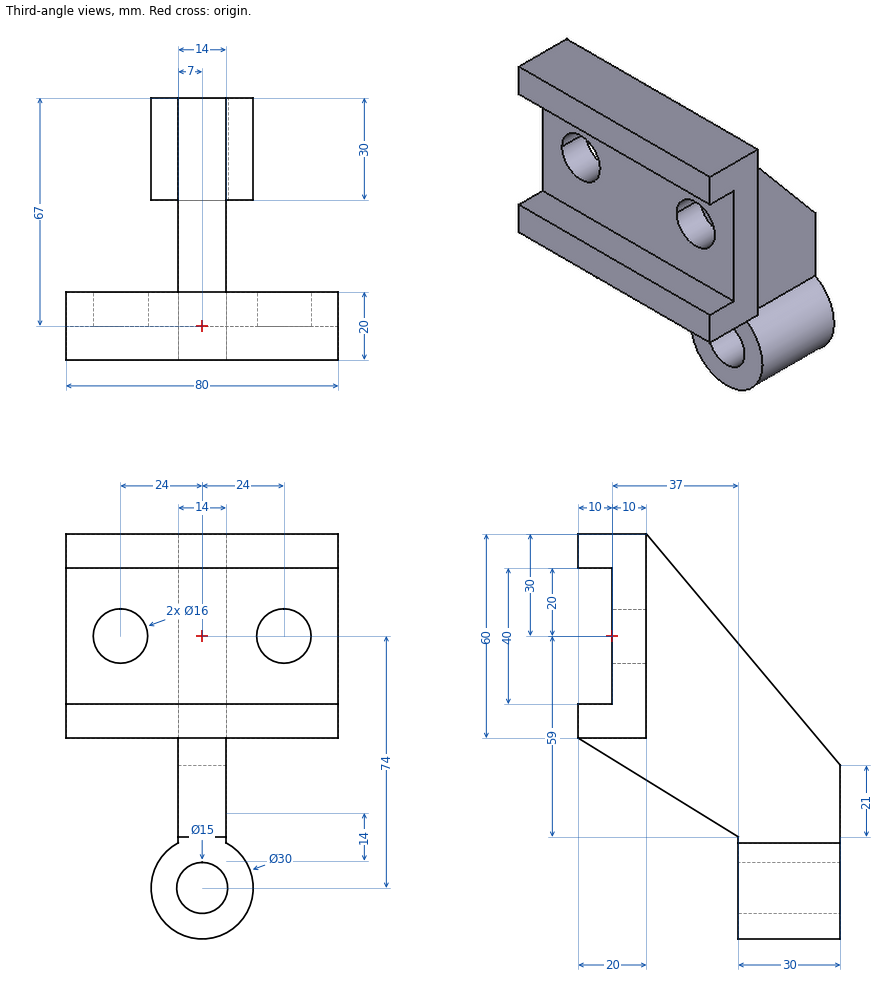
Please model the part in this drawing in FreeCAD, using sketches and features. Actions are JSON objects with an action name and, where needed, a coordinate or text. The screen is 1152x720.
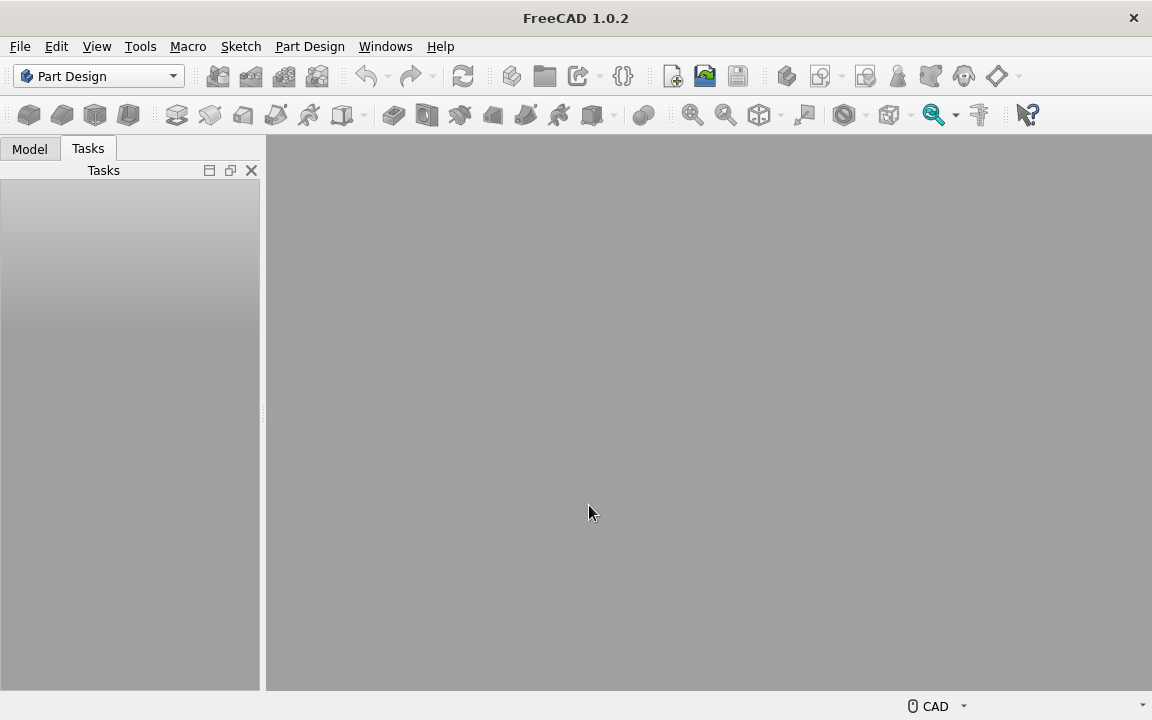
{"action": "left_click", "coordinate": [672, 76]}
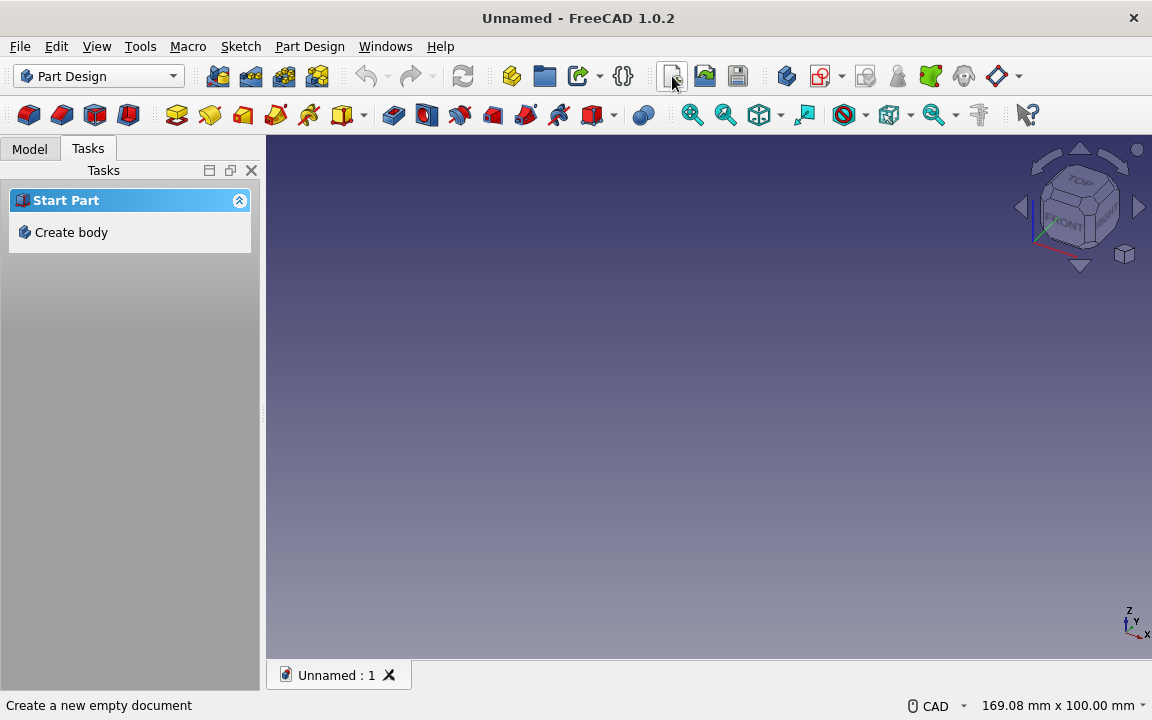
{"action": "left_click", "coordinate": [820, 76]}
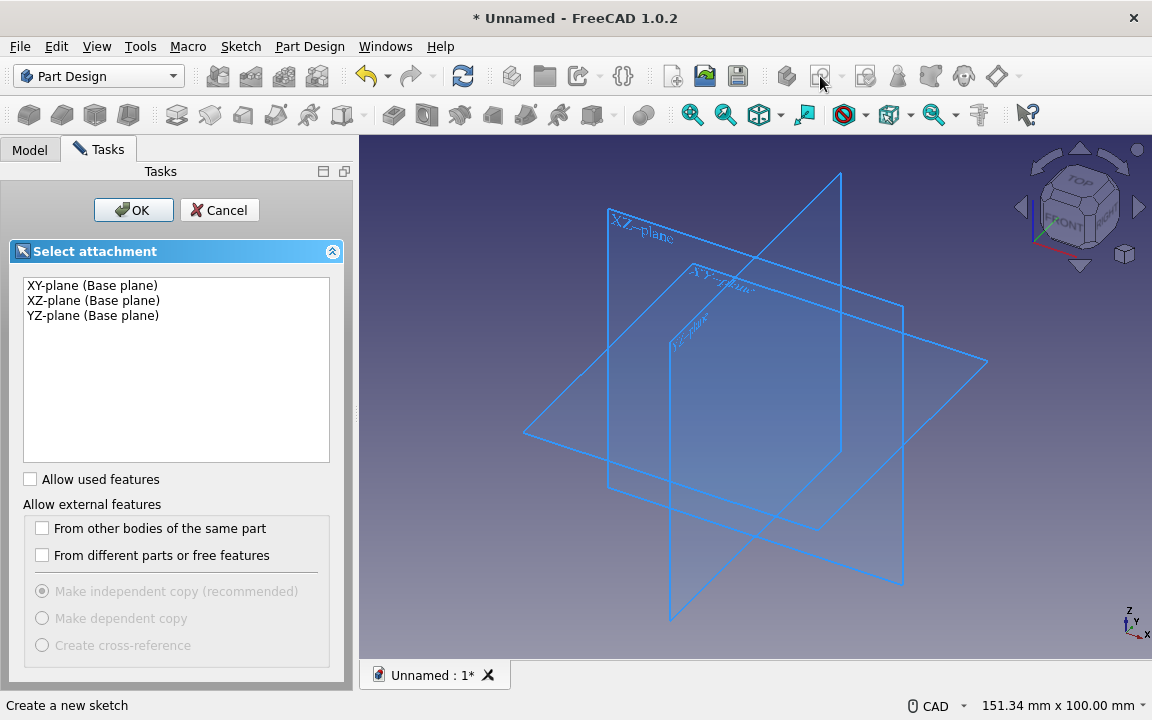
{"action": "left_click", "coordinate": [84, 286]}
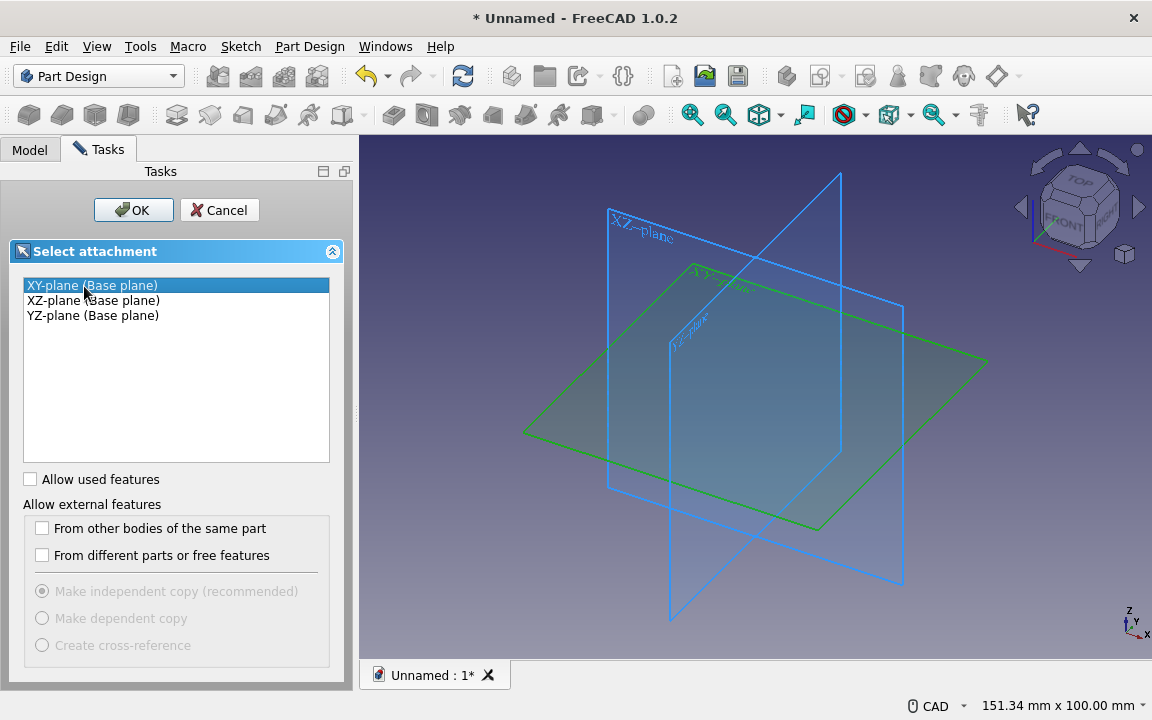
{"action": "left_click", "coordinate": [134, 210]}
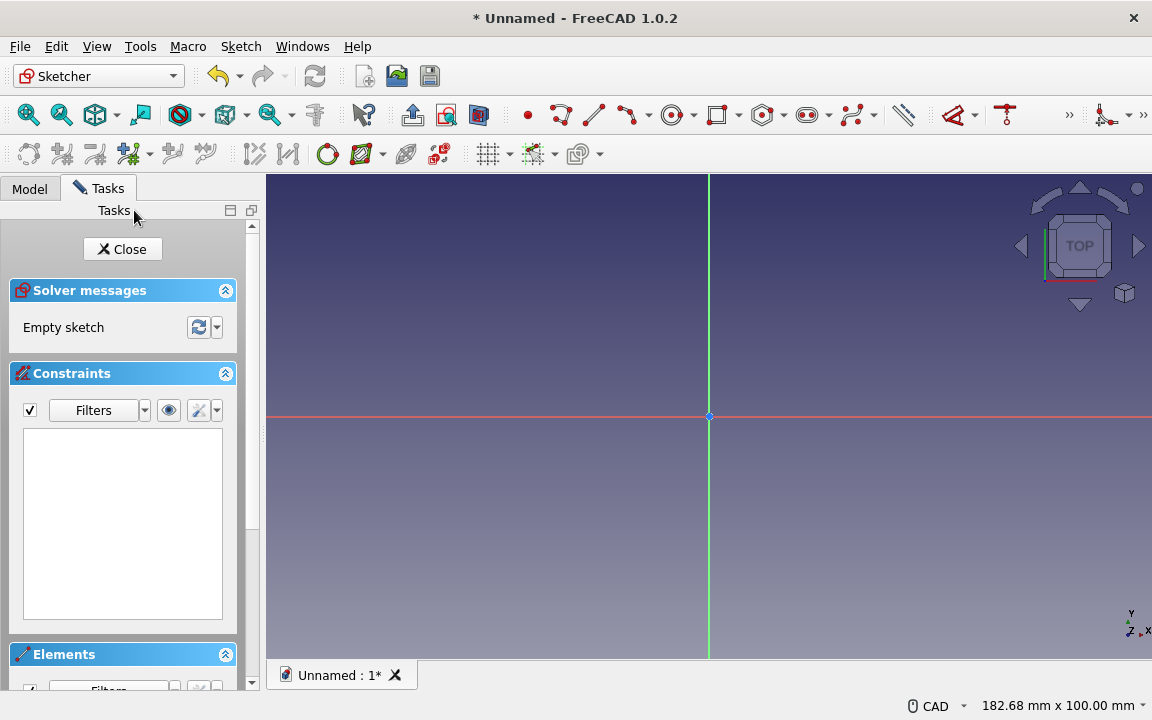
{"action": "left_click", "coordinate": [738, 116]}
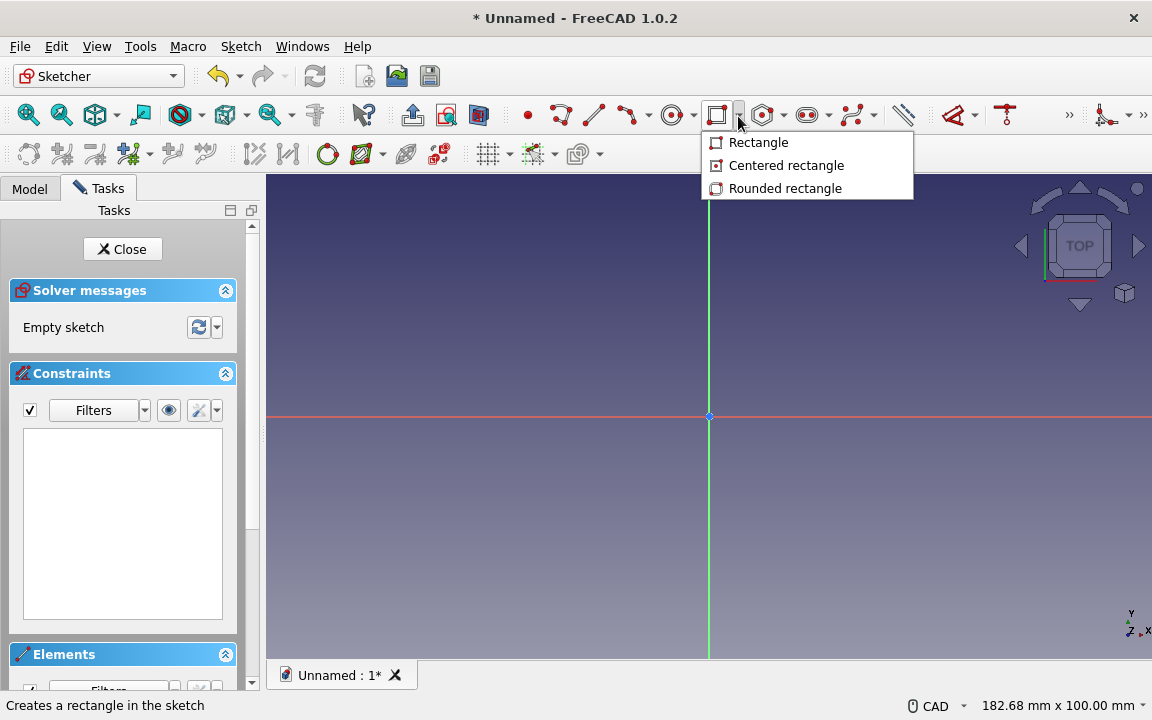
{"action": "left_click", "coordinate": [808, 166]}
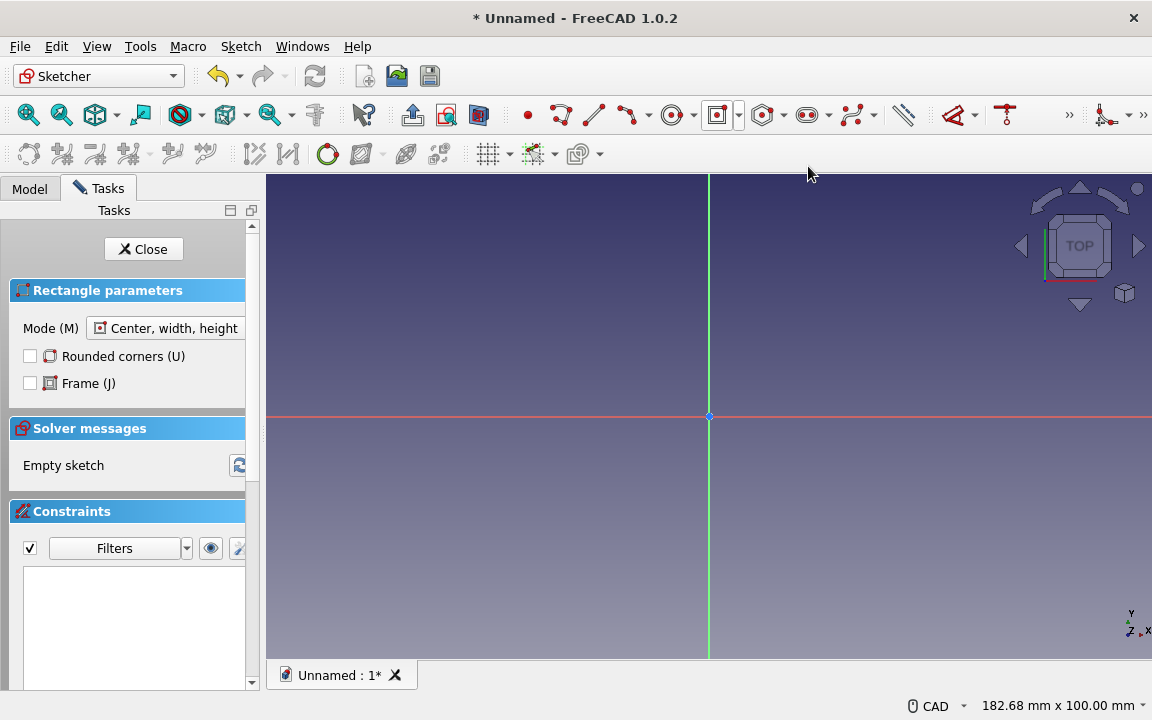
{"action": "left_click", "coordinate": [709, 416]}
{"action": "mouse_move", "coordinate": [903, 368]}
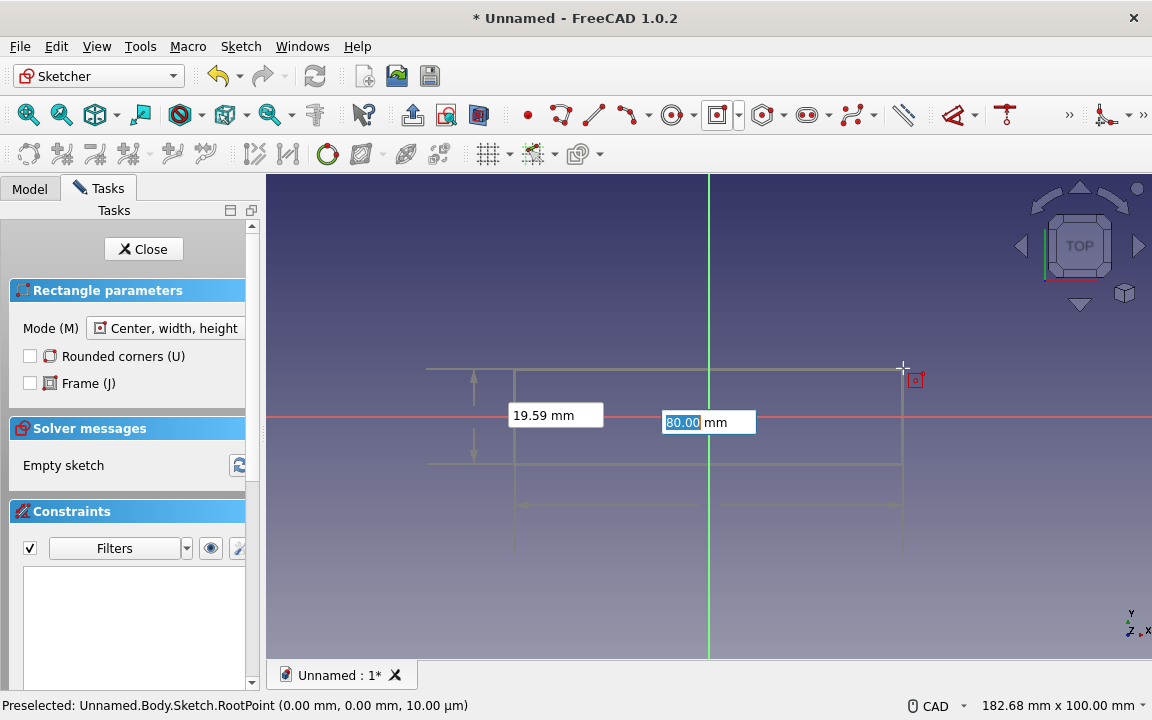
{"action": "type", "text": "80"}
{"action": "key", "text": "Tab"}
{"action": "type", "text": "20"}
{"action": "key", "text": "Return"}
{"action": "key", "text": "Escape"}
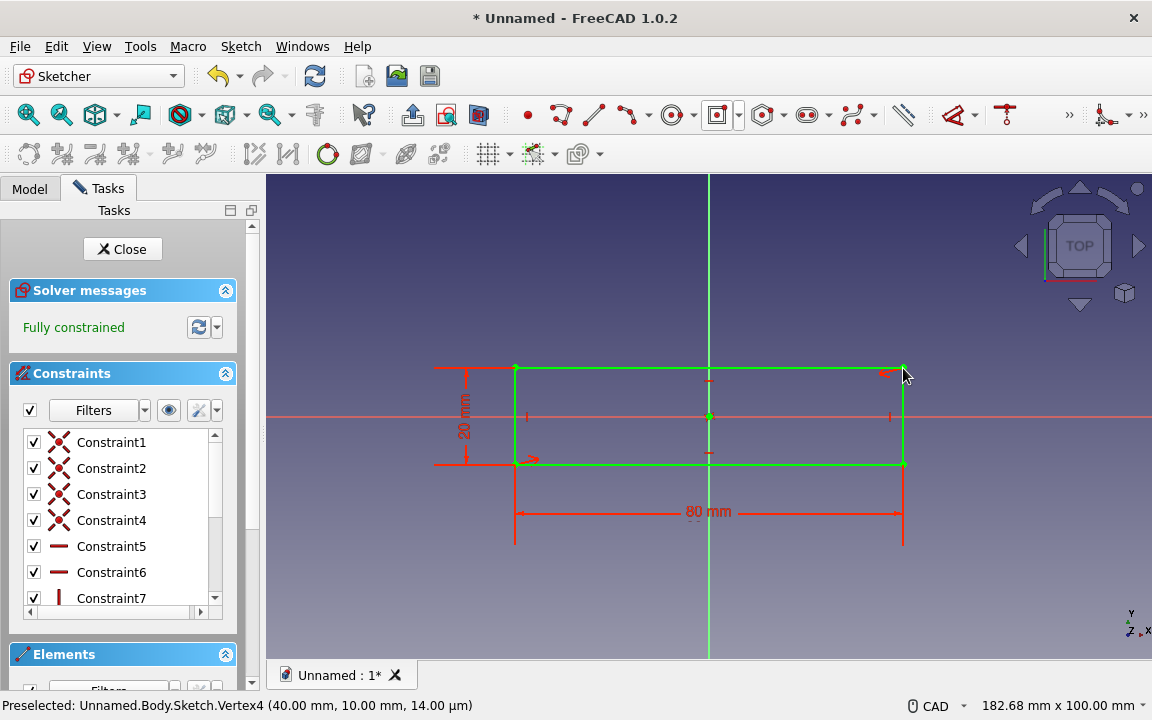
{"action": "left_click", "coordinate": [123, 249]}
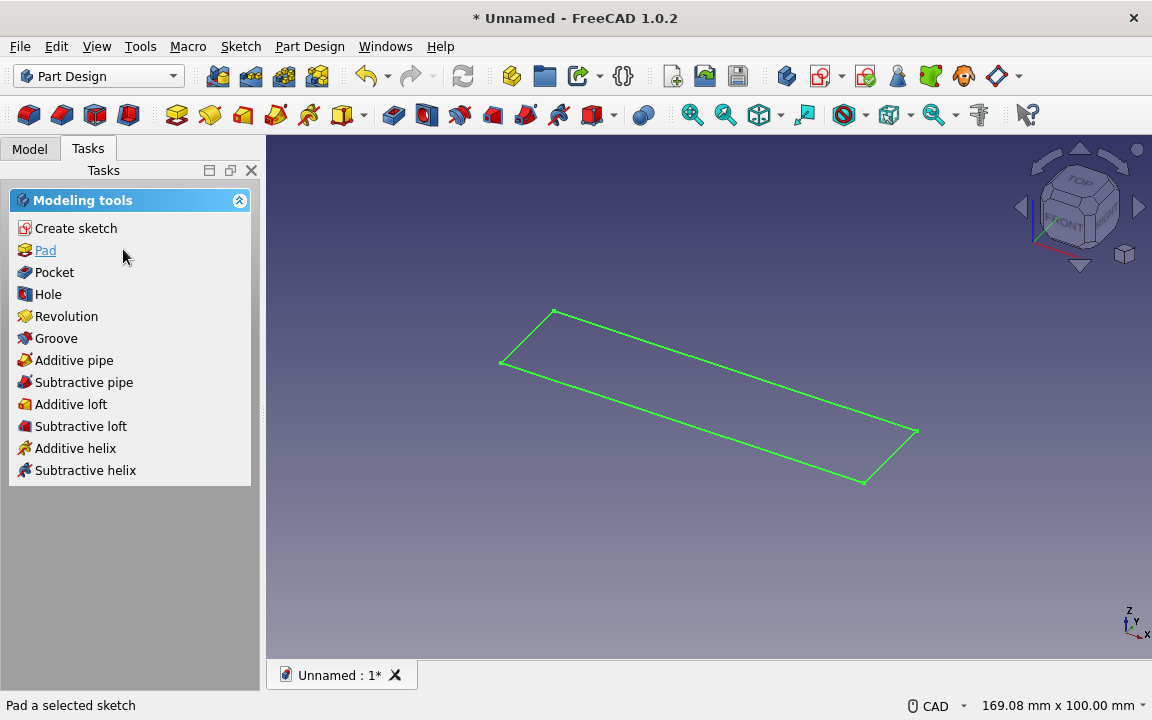
{"action": "left_click", "coordinate": [177, 116]}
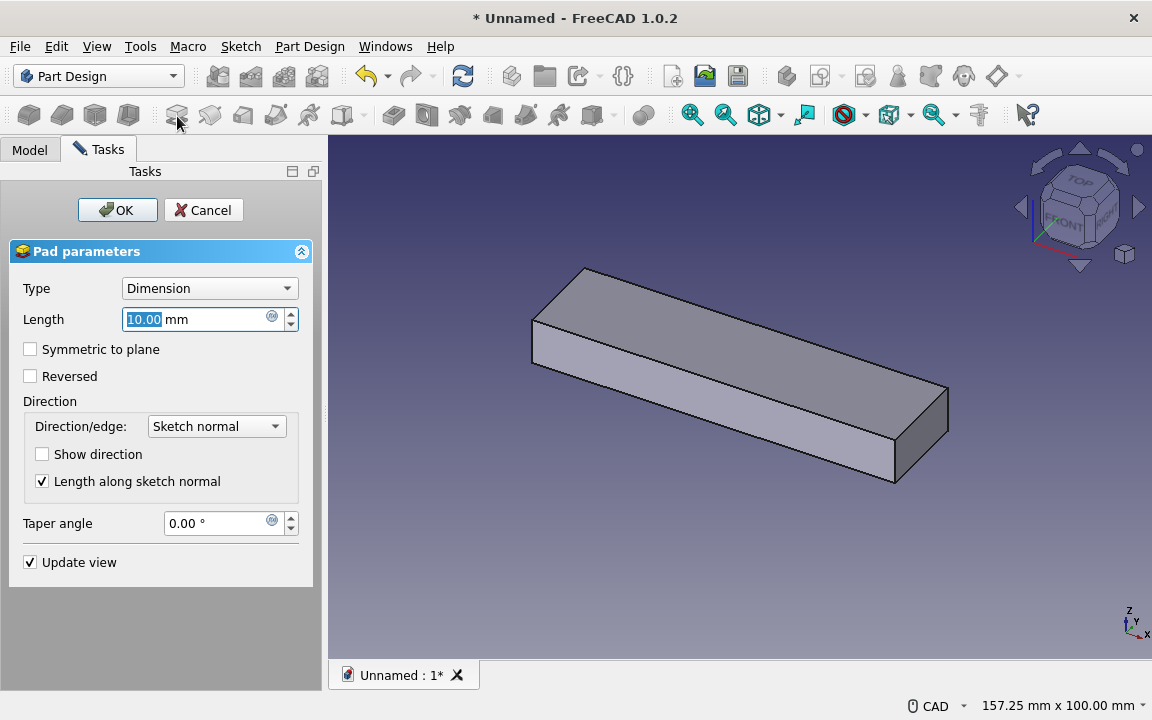
{"action": "type", "text": "60"}
{"action": "key", "text": "Tab"}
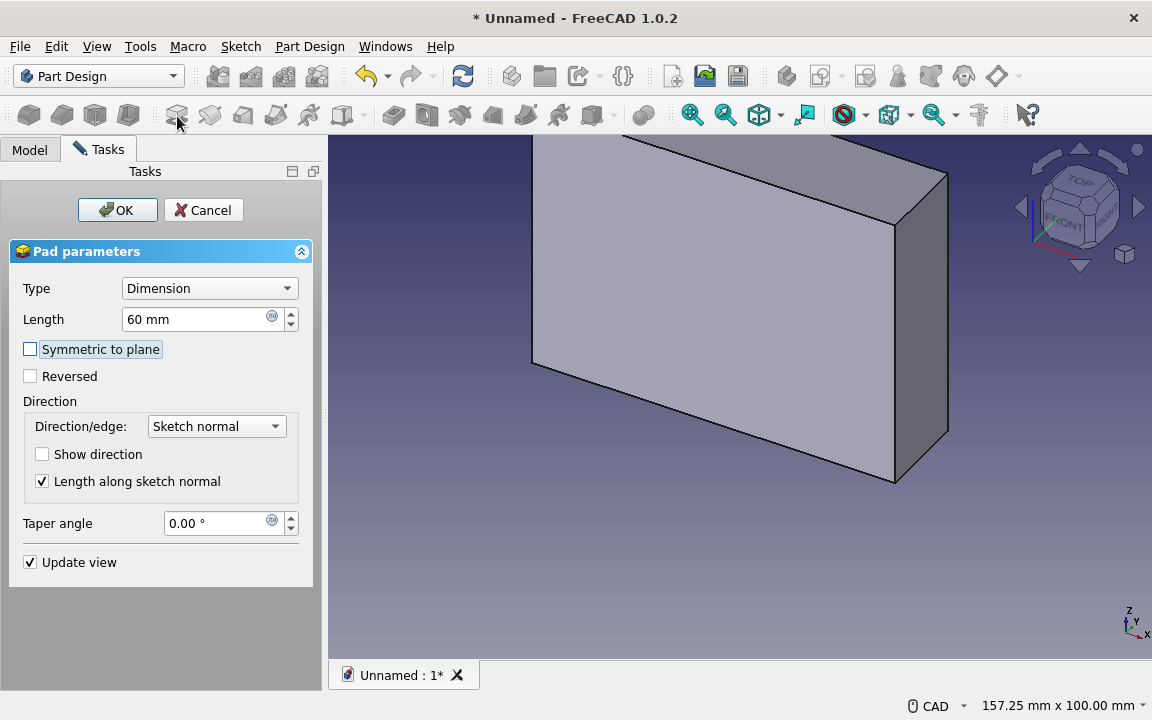
{"action": "left_click", "coordinate": [31, 349]}